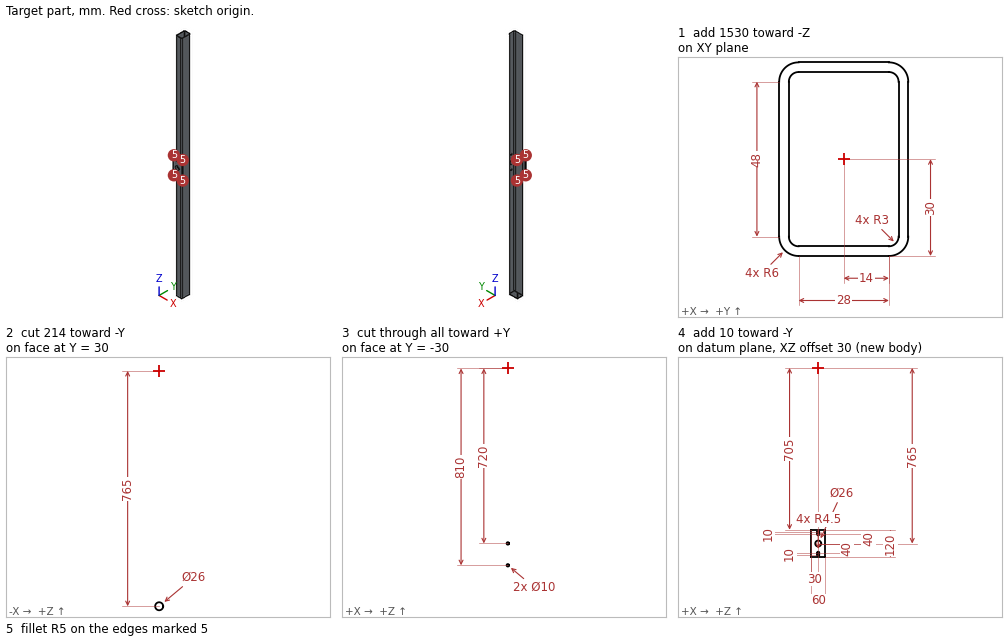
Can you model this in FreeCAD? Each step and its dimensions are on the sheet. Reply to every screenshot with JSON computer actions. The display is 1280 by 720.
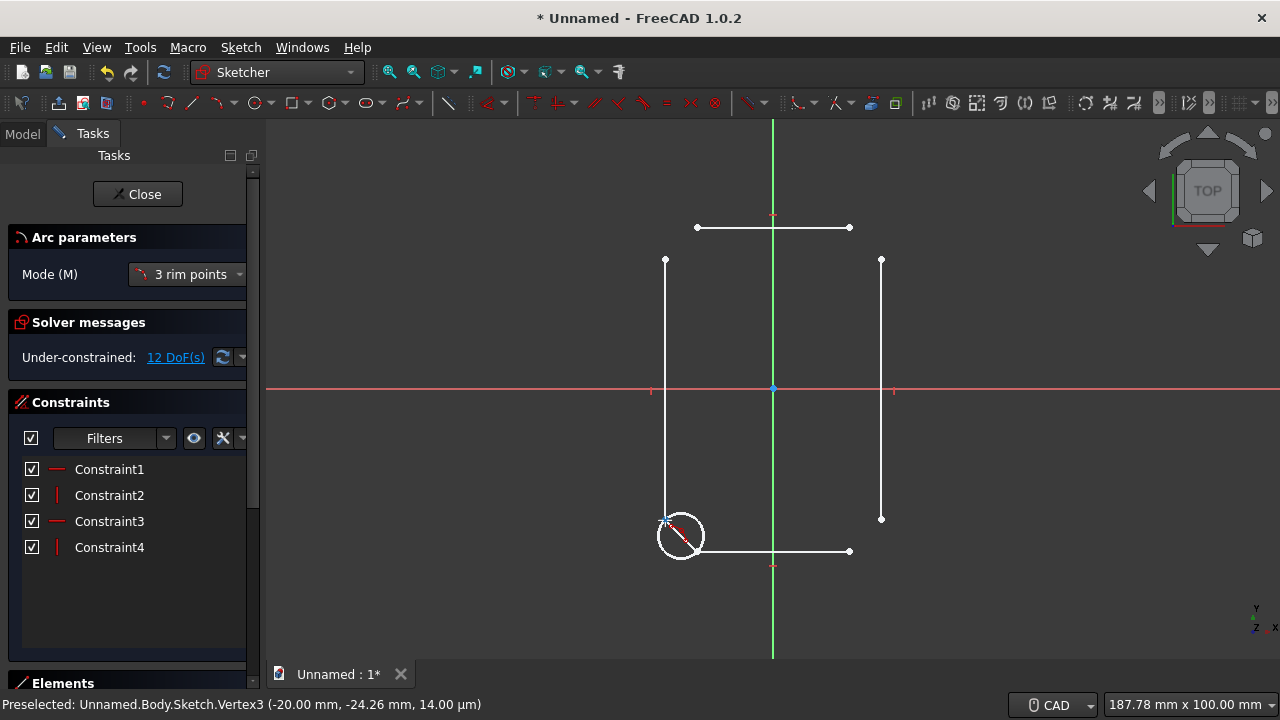
{"action": "scroll", "coordinate": [674, 542], "scroll_direction": "up", "scroll_amount": 3}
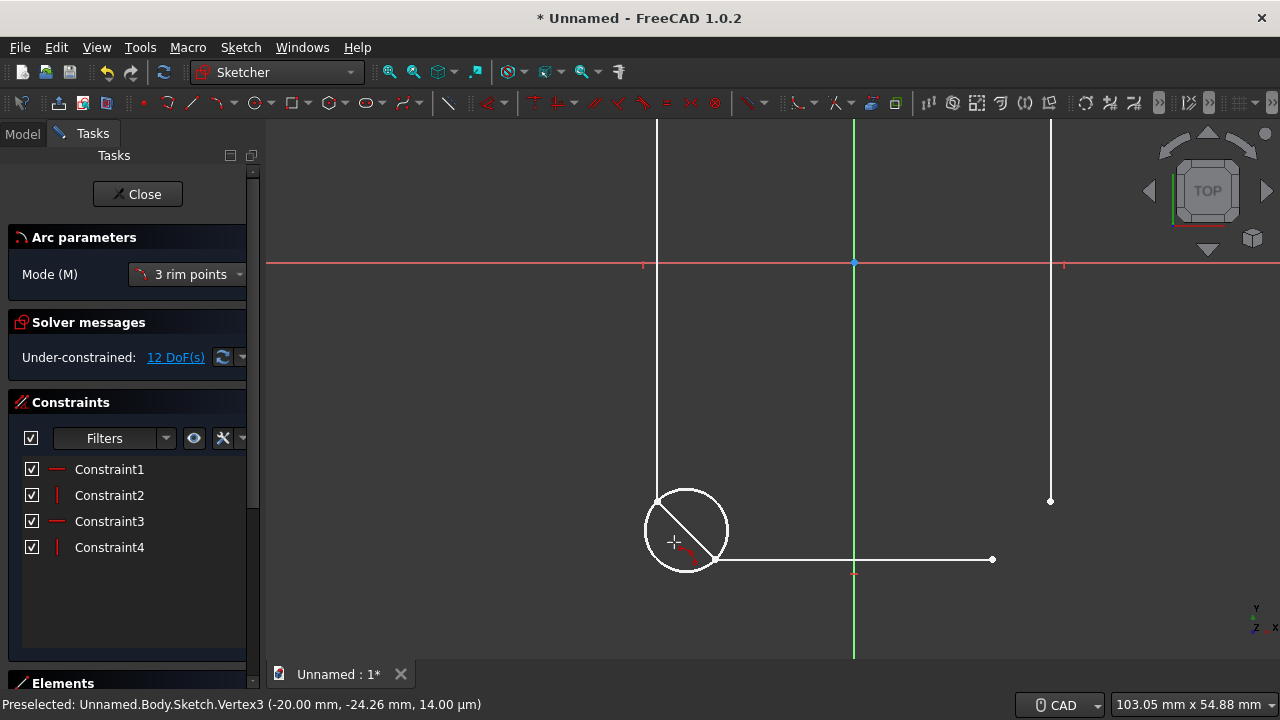
{"action": "left_click", "coordinate": [675, 540]}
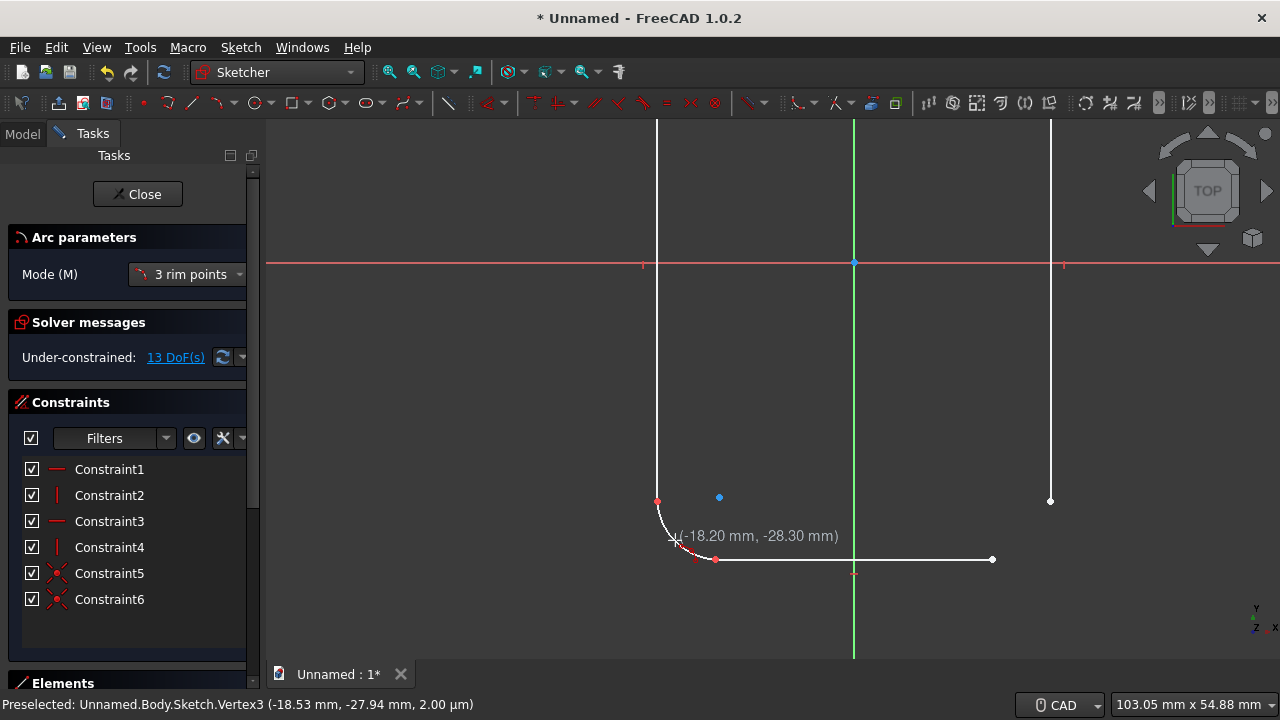
{"action": "scroll", "coordinate": [523, 543], "scroll_direction": "down", "scroll_amount": 3}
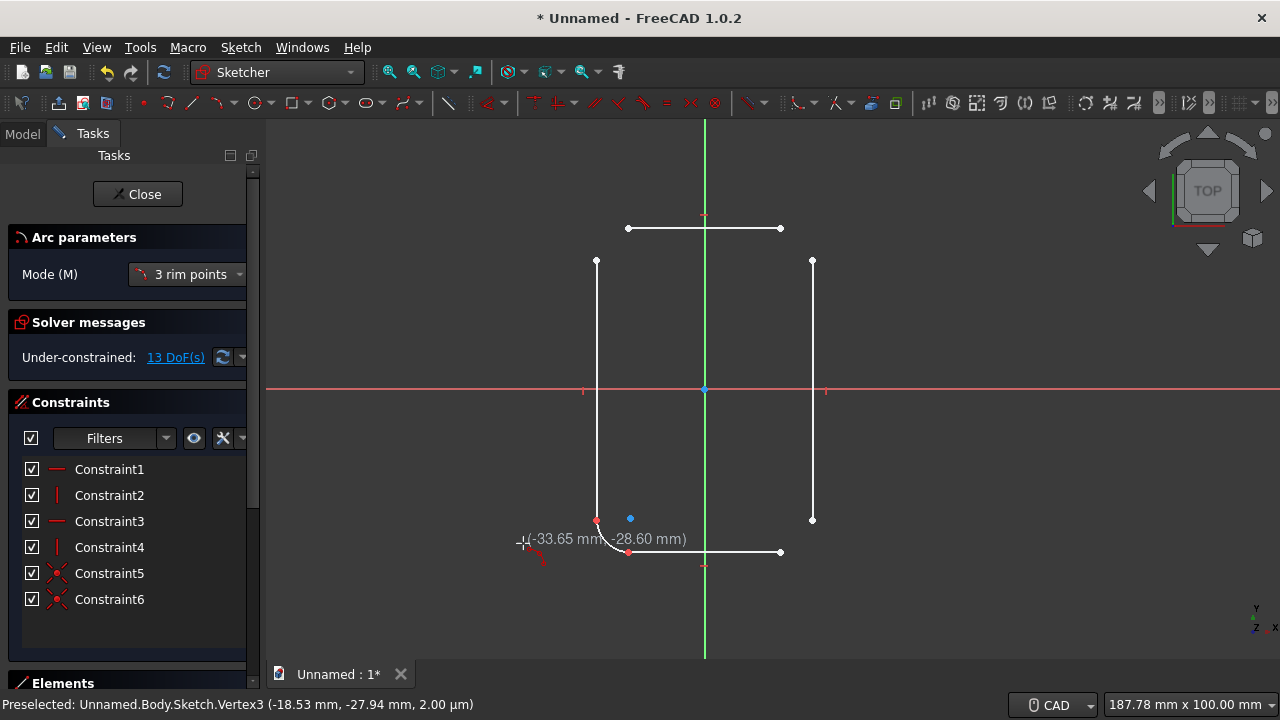
{"action": "left_click", "coordinate": [597, 260]}
{"action": "left_click", "coordinate": [629, 228]}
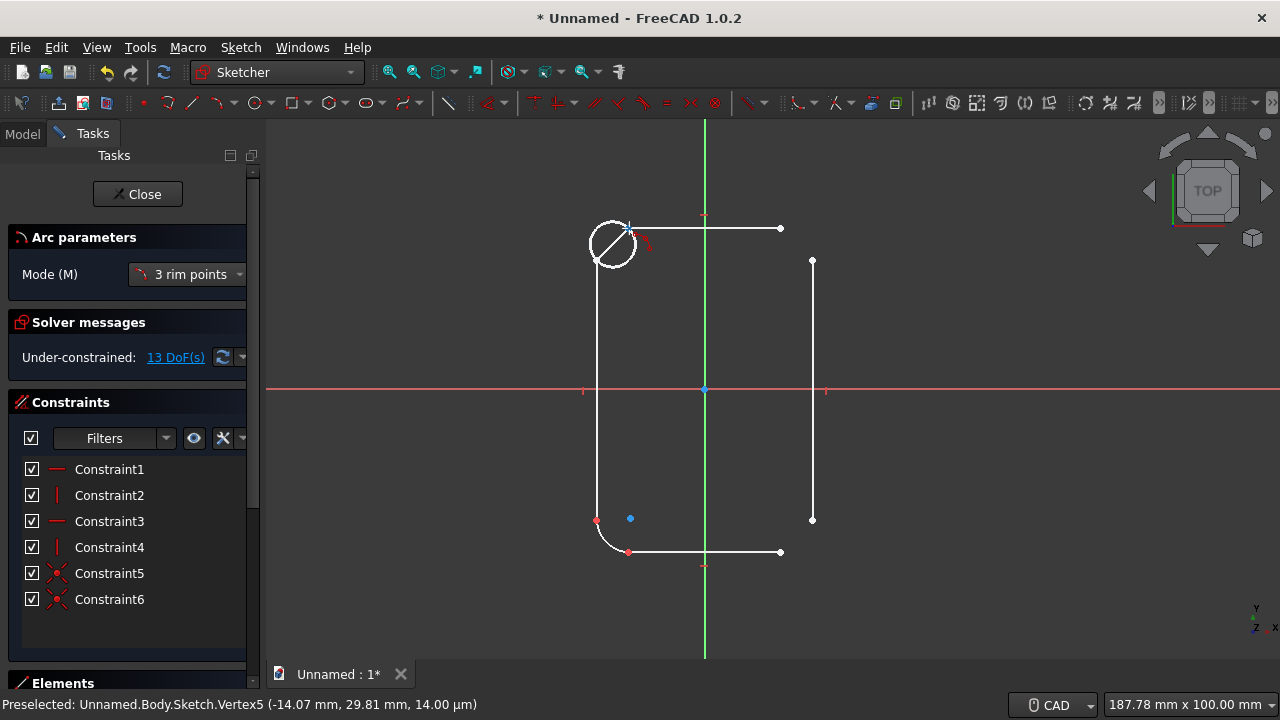
{"action": "scroll", "coordinate": [606, 237], "scroll_direction": "up", "scroll_amount": 3}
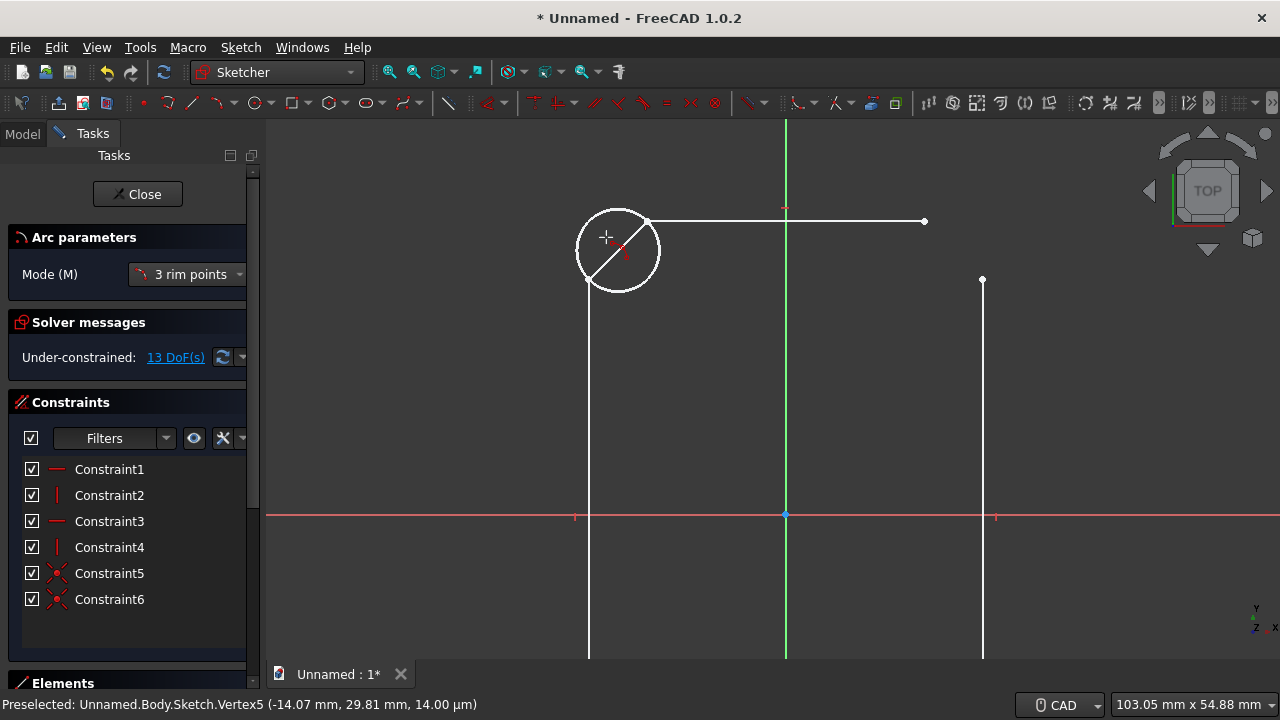
{"action": "left_click", "coordinate": [606, 237]}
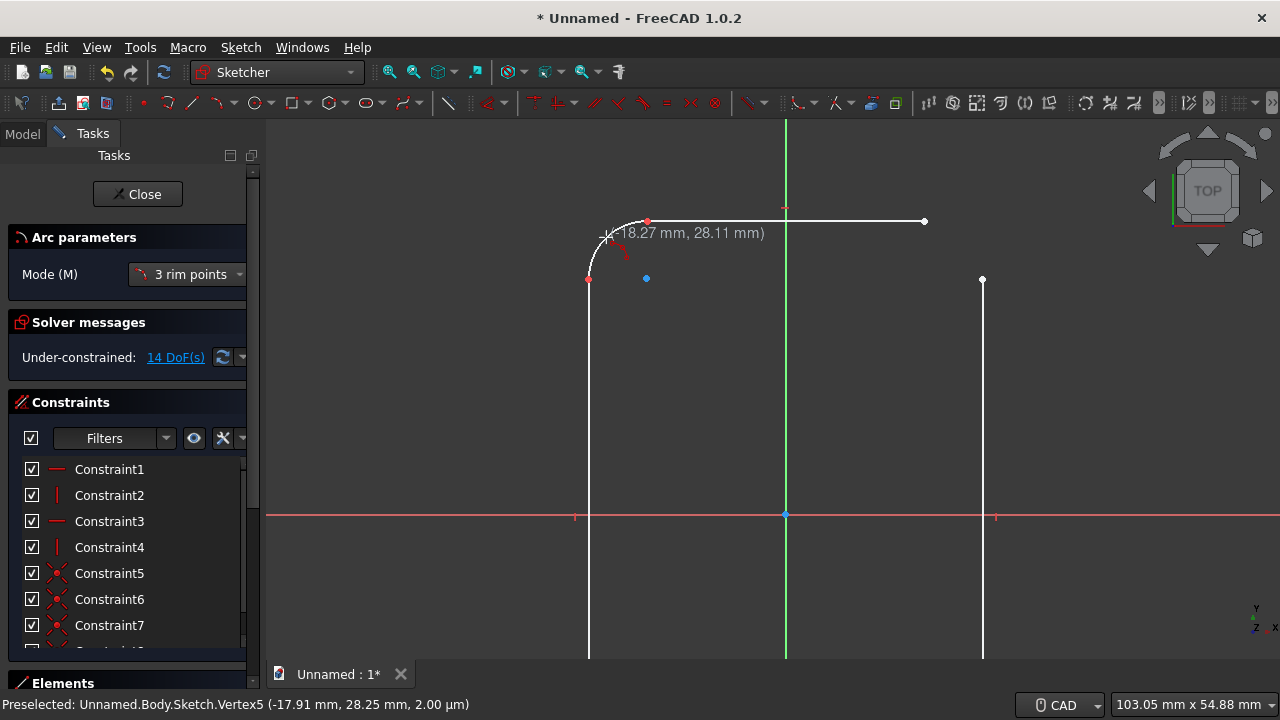
{"action": "left_click", "coordinate": [924, 221]}
{"action": "left_click", "coordinate": [983, 280]}
{"action": "left_click", "coordinate": [965, 237]}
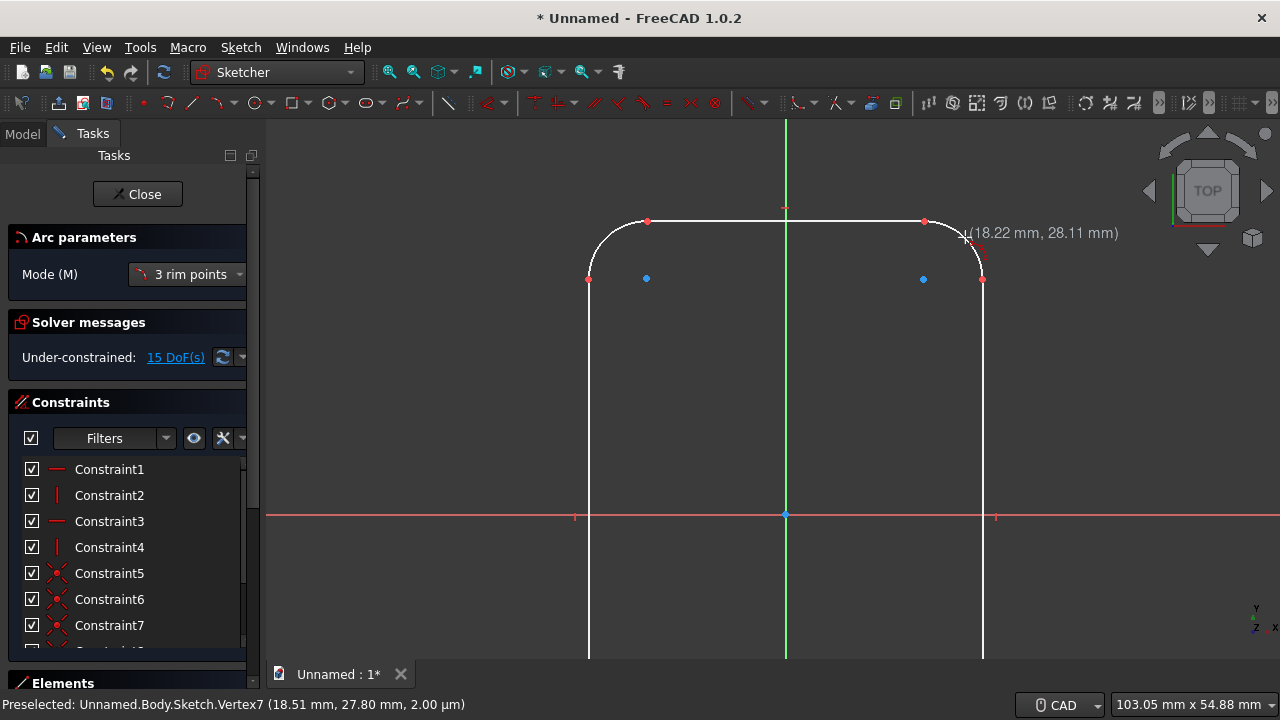
{"action": "scroll", "coordinate": [606, 236], "scroll_direction": "down", "scroll_amount": 3}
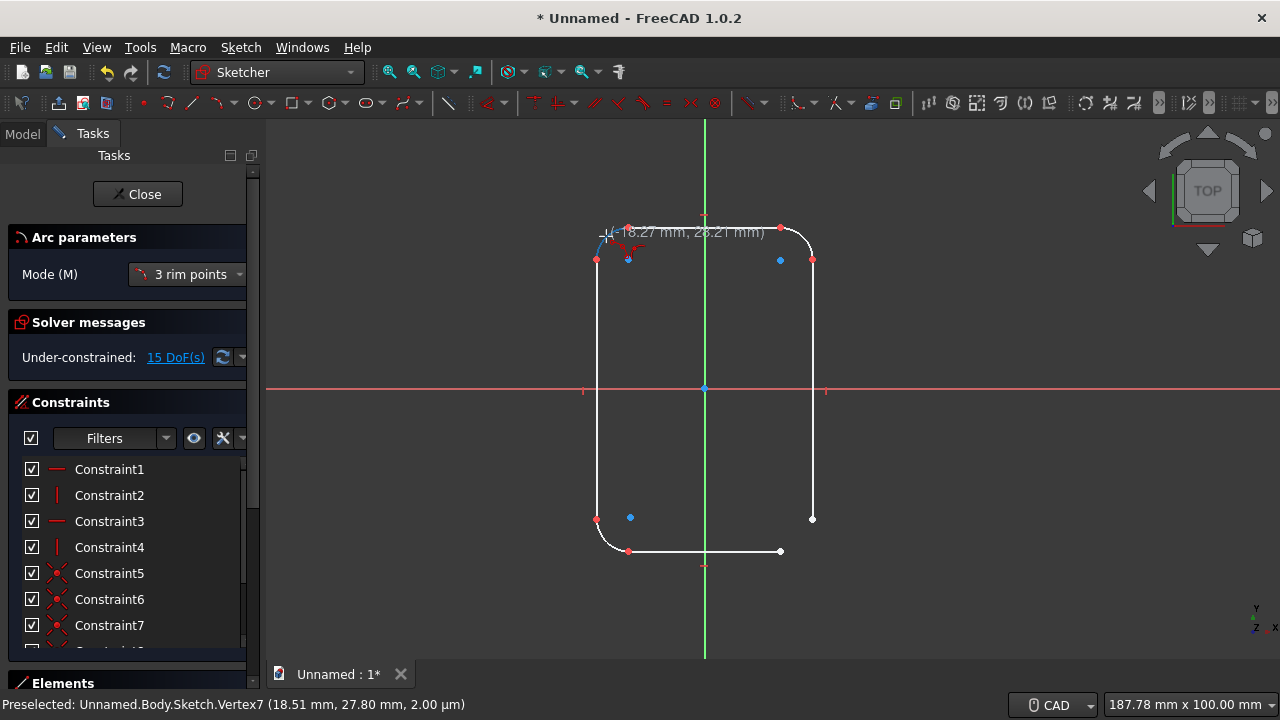
{"action": "left_click", "coordinate": [813, 520]}
{"action": "left_click", "coordinate": [781, 552]}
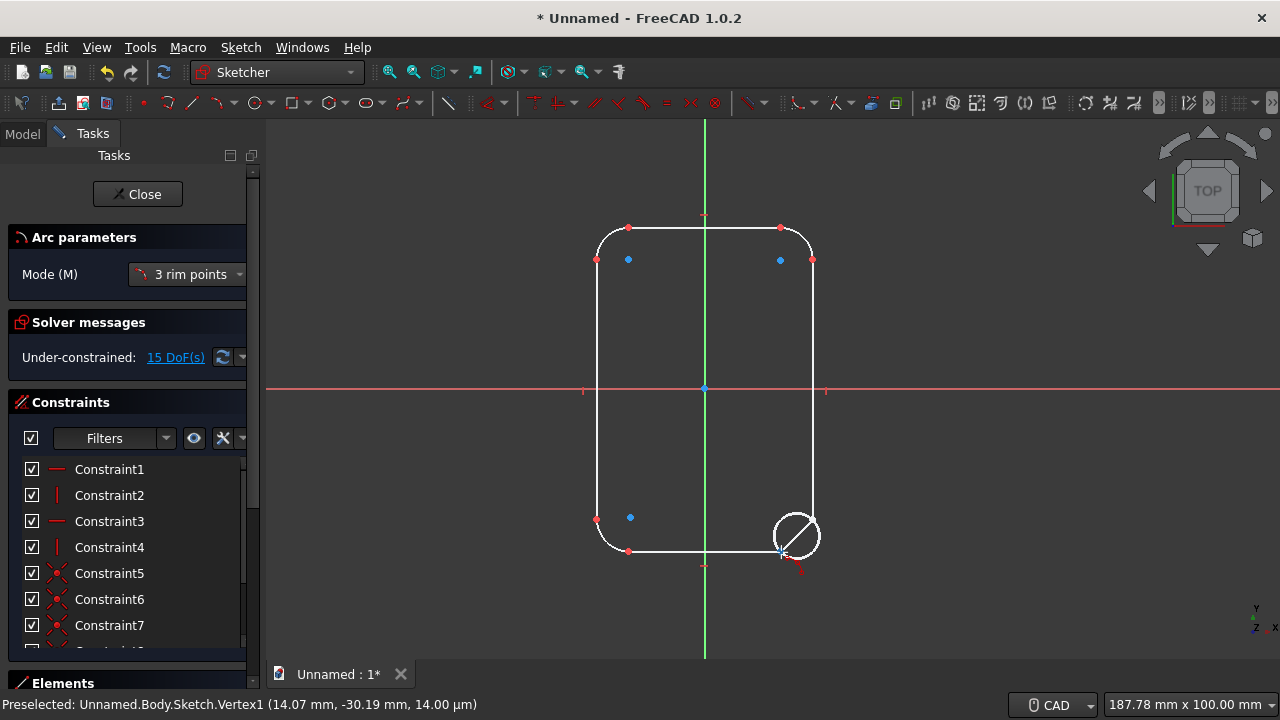
{"action": "scroll", "coordinate": [803, 542], "scroll_direction": "up", "scroll_amount": 3}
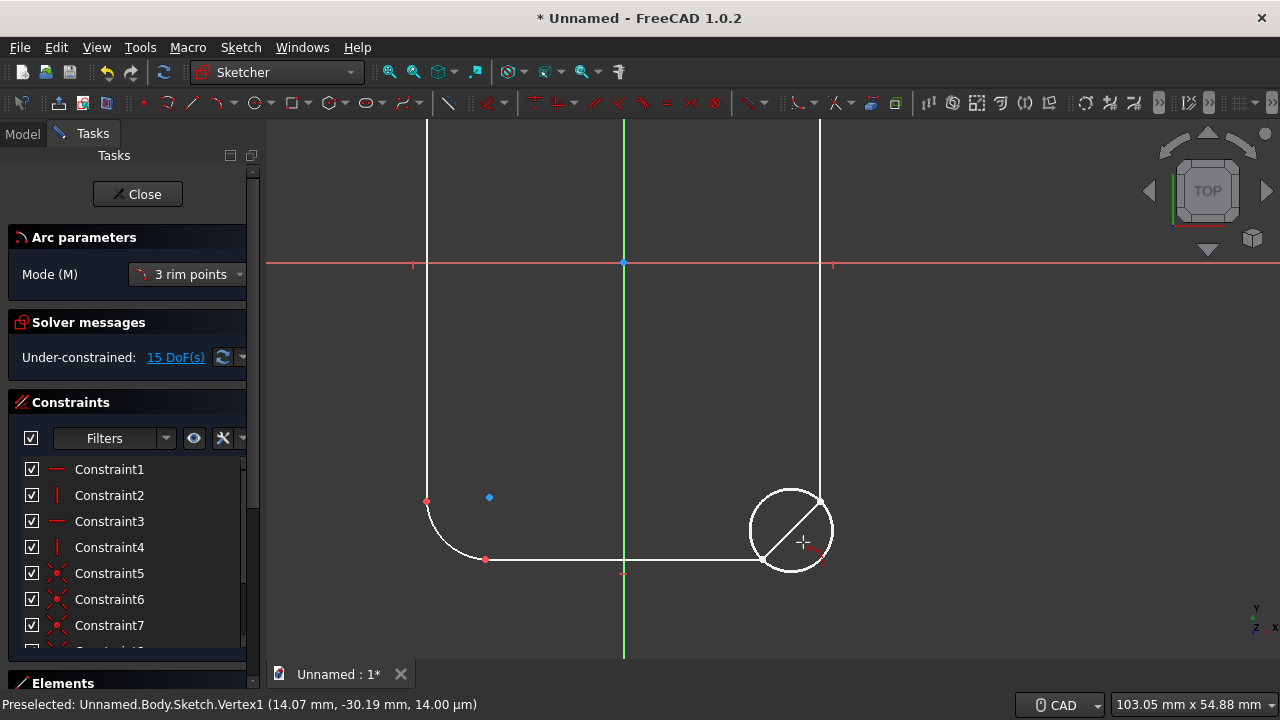
{"action": "left_click", "coordinate": [803, 540]}